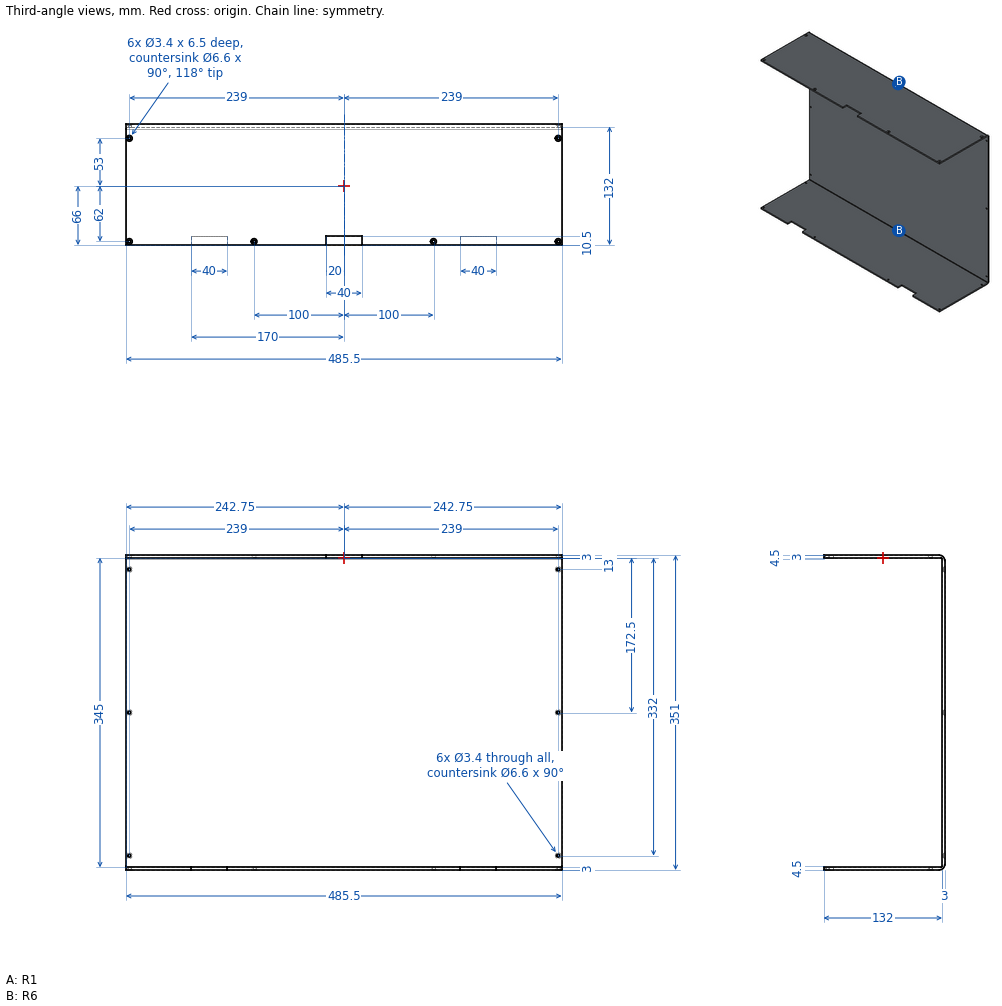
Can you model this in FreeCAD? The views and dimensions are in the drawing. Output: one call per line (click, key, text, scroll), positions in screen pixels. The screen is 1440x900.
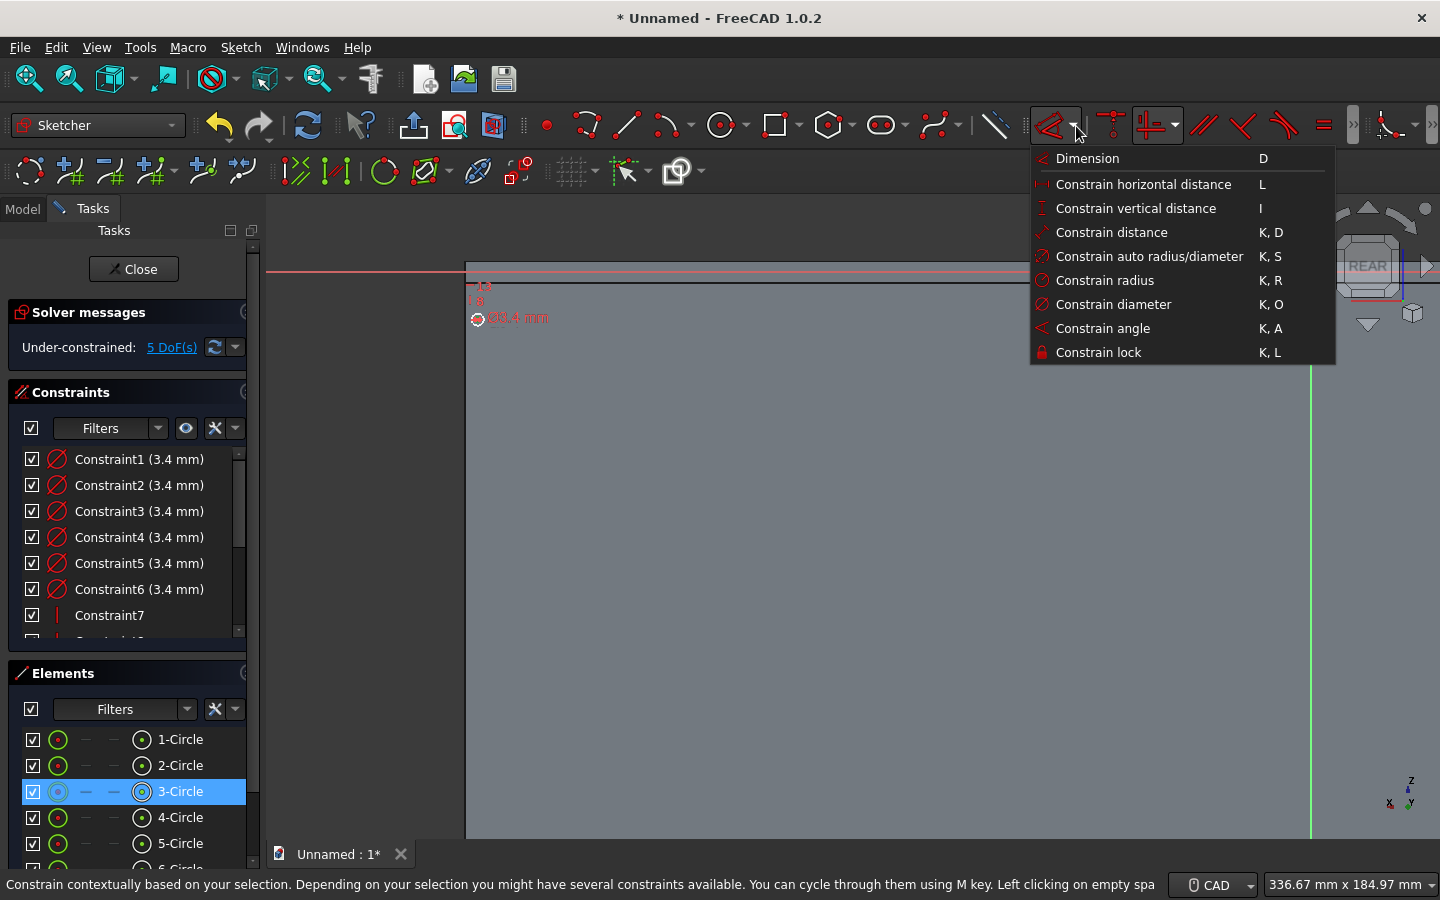
click(1183, 208)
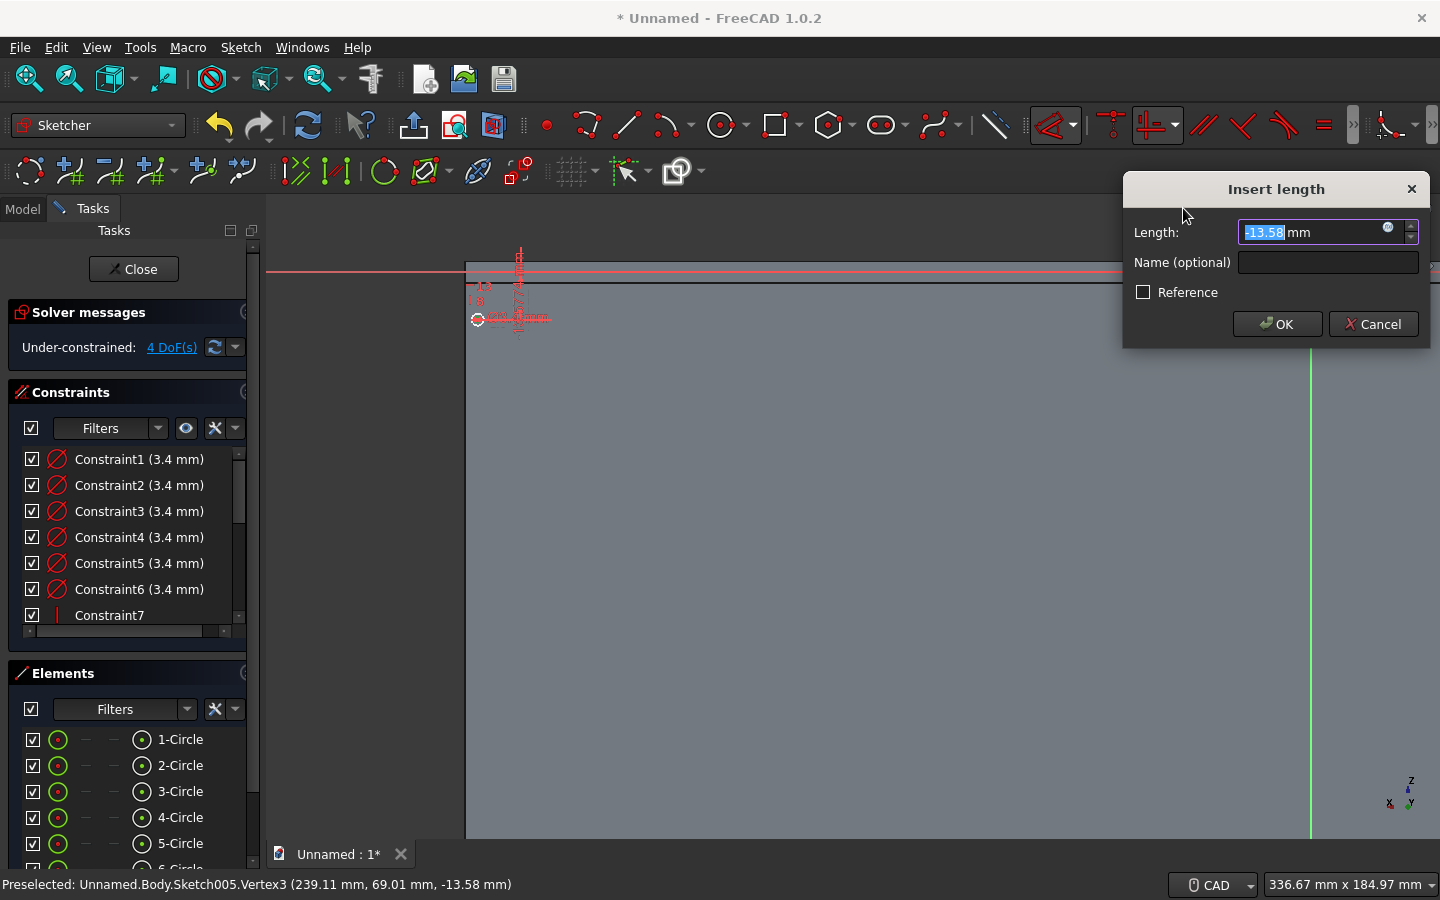
text(-13)
key(Return)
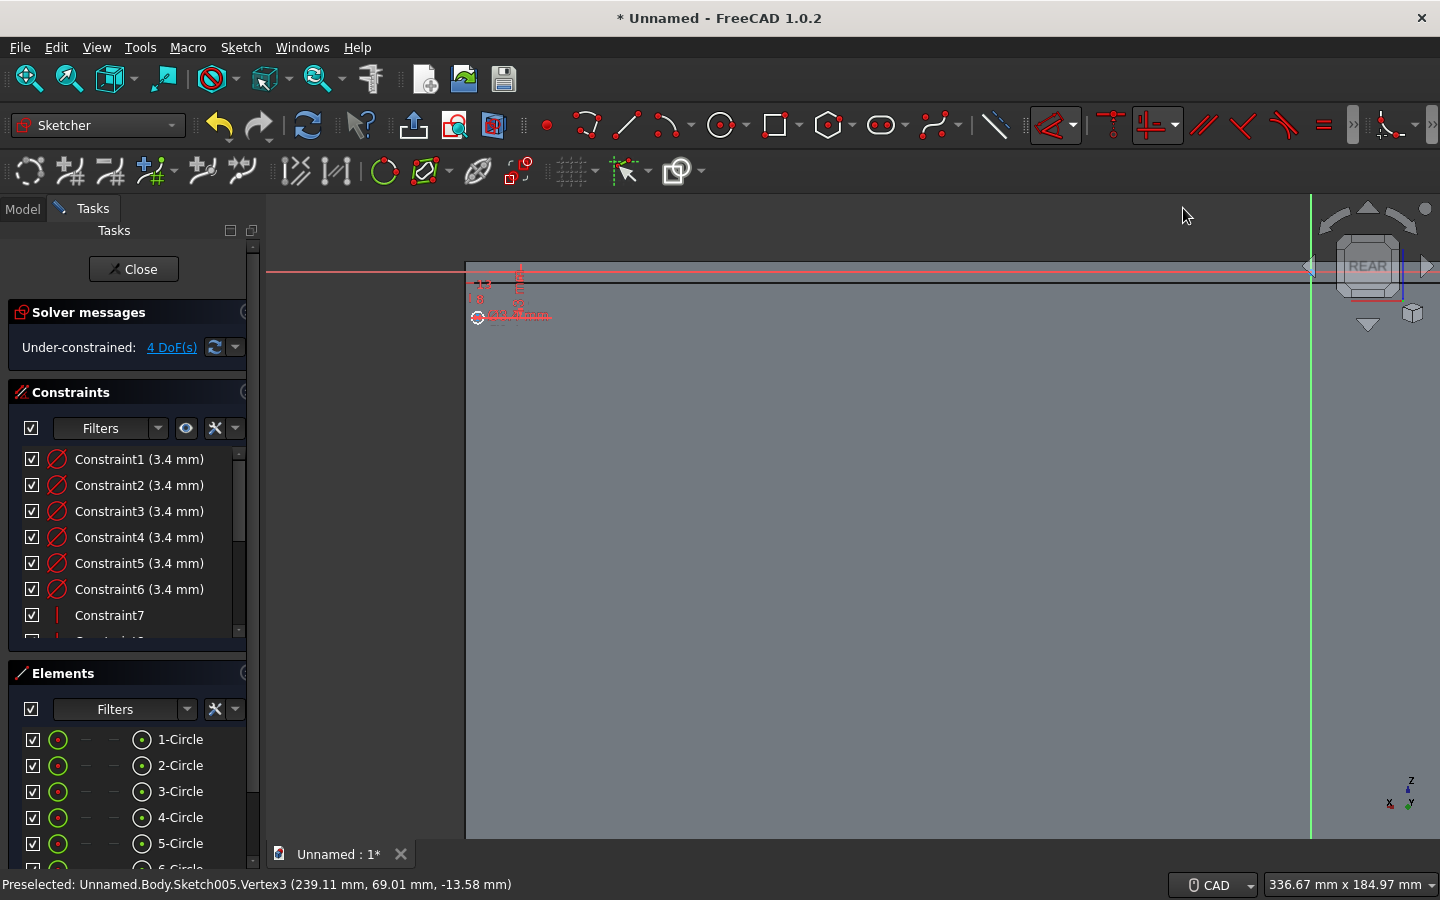
scroll(478, 320, down, 5)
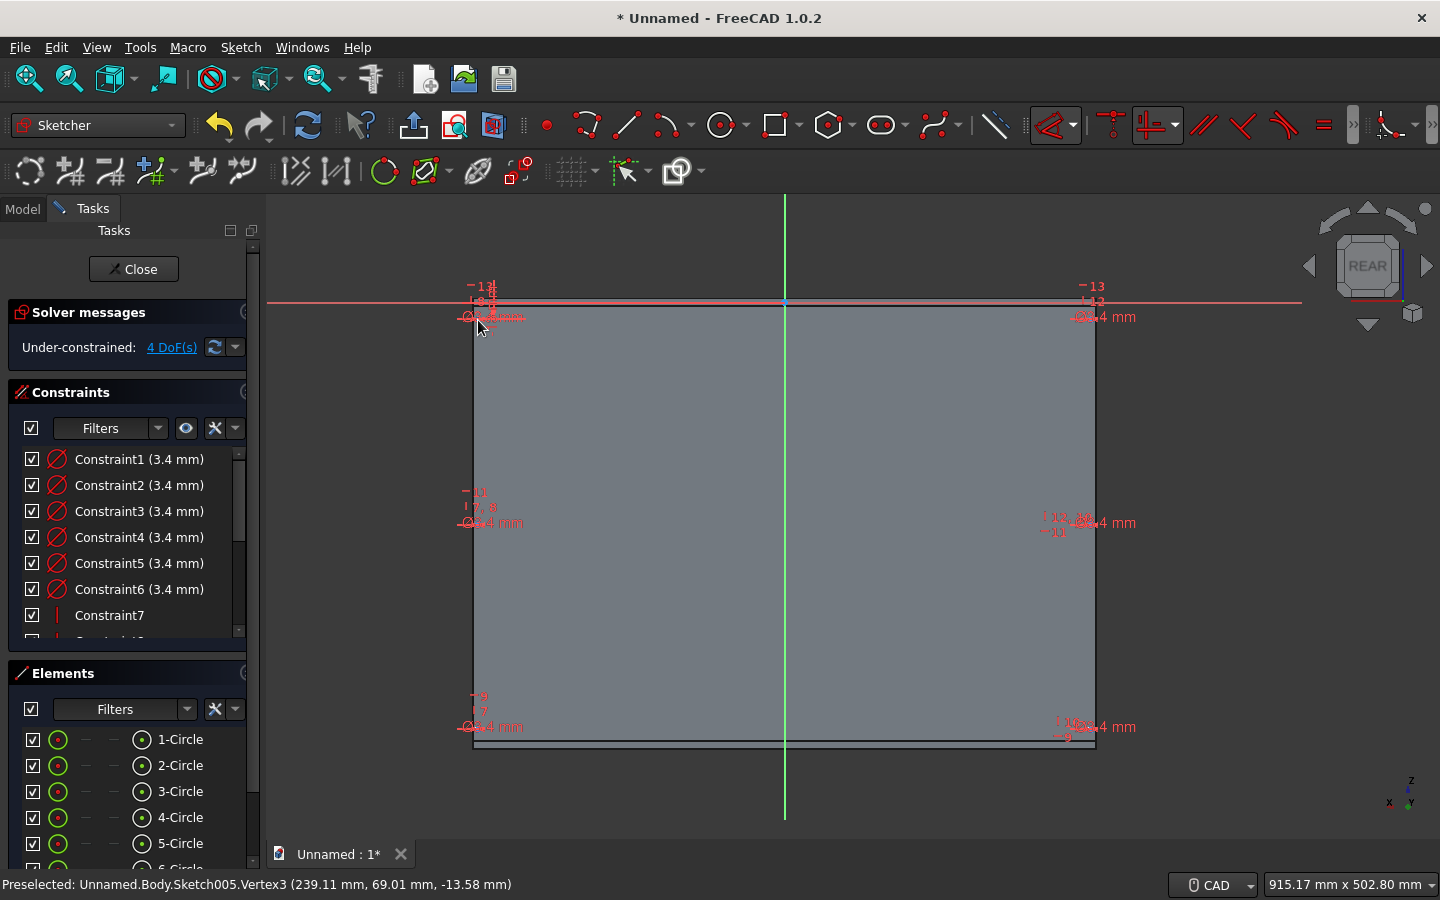
click(478, 729)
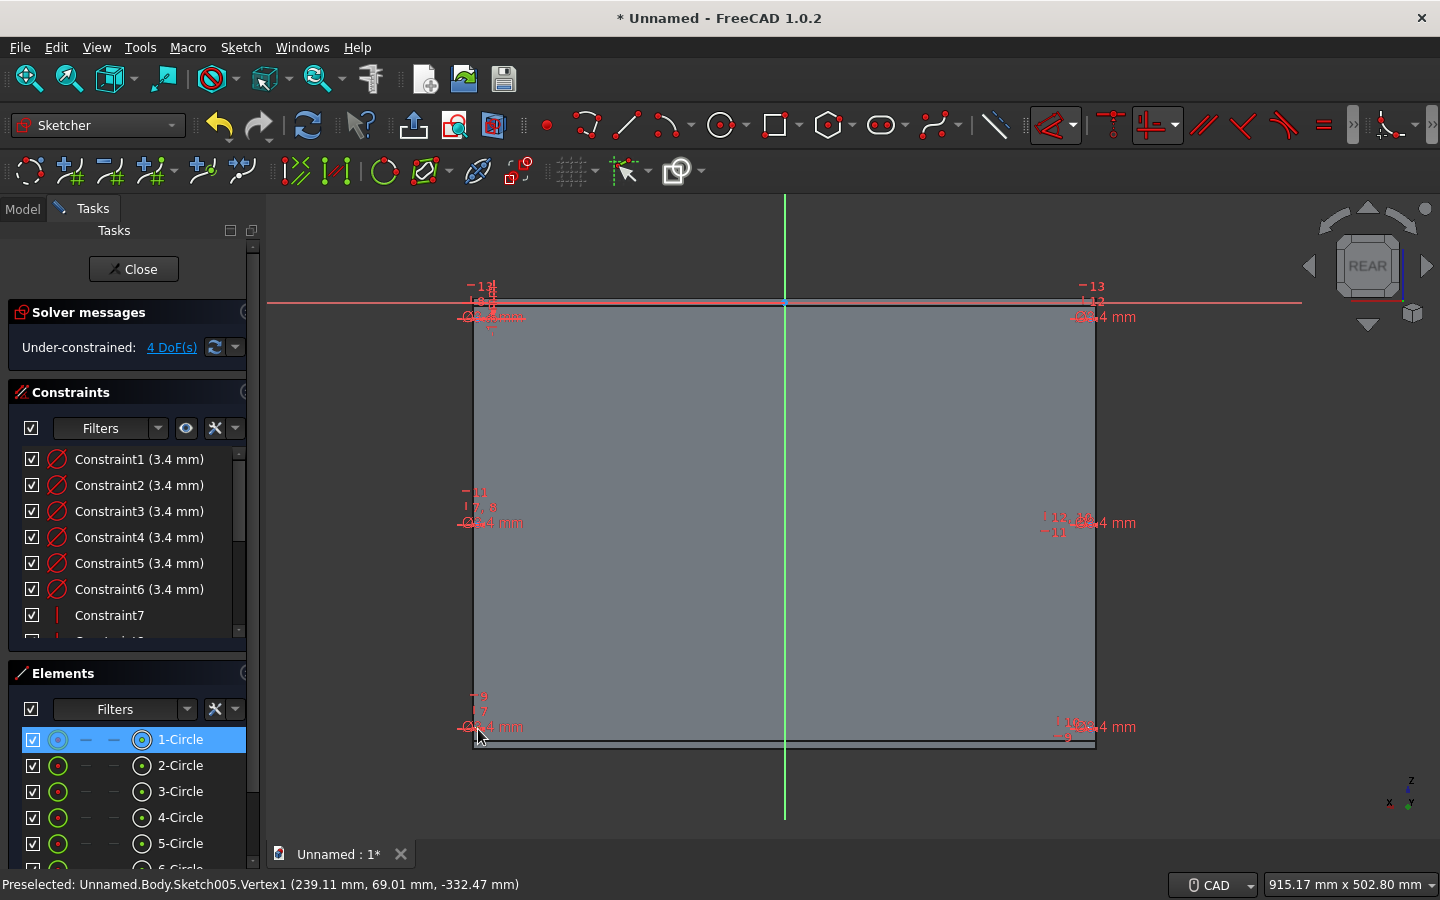
key(l)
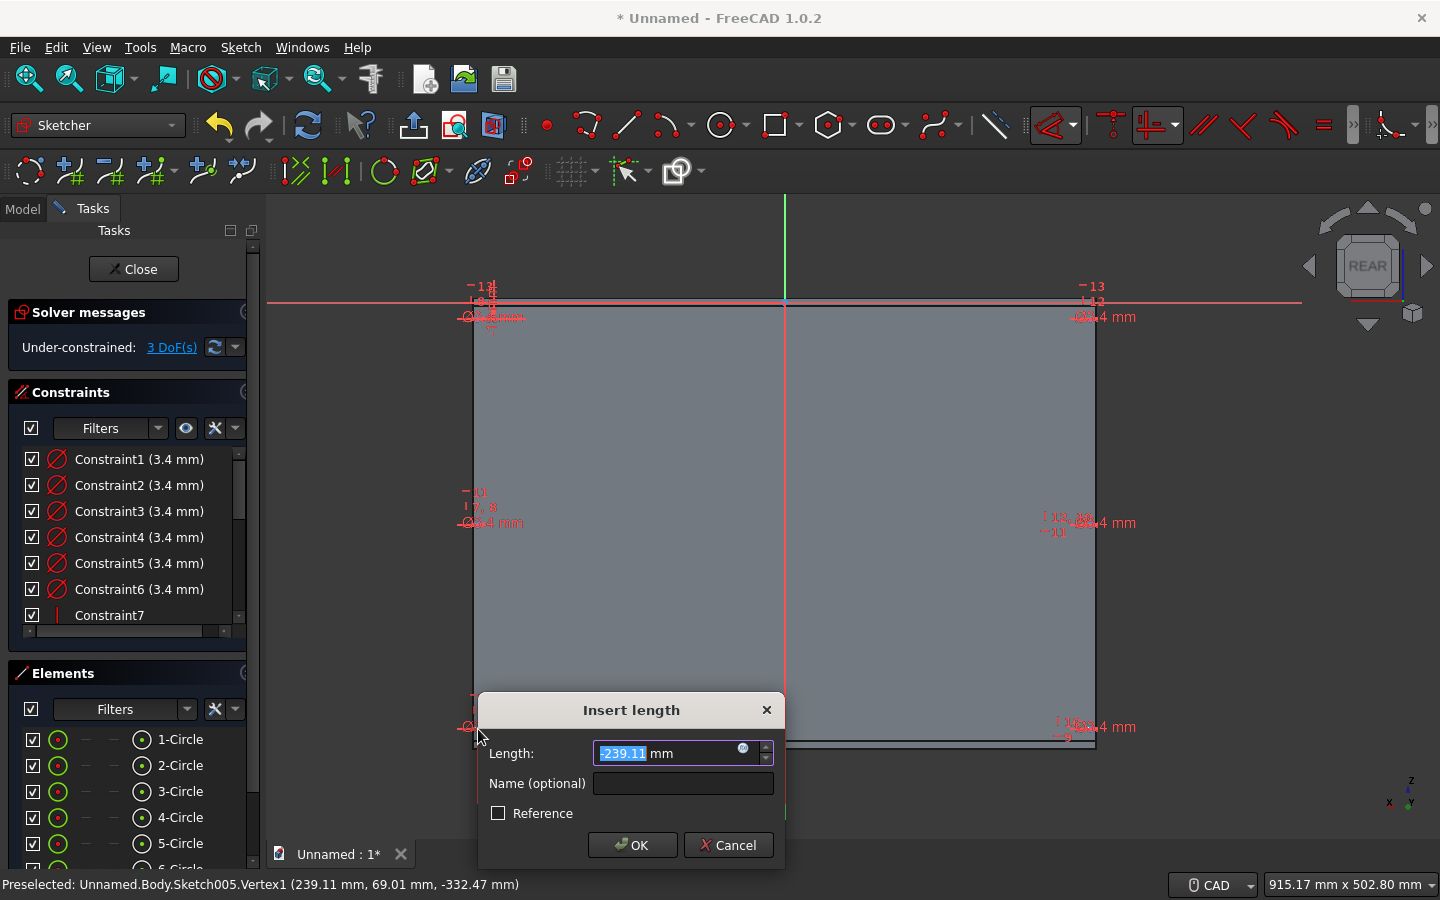
text(-239)
key(Return)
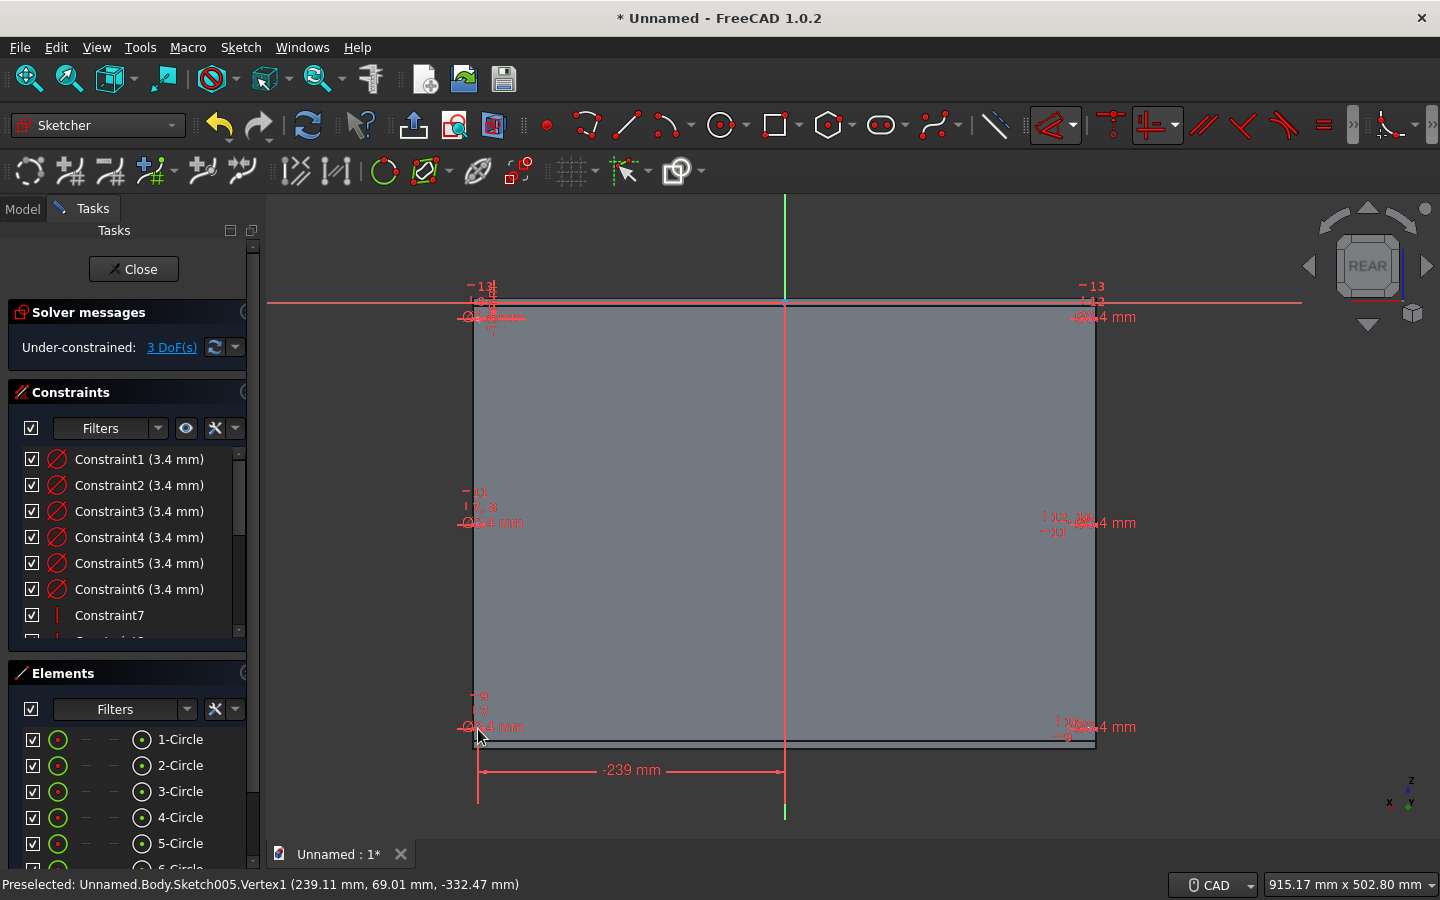
click(478, 729)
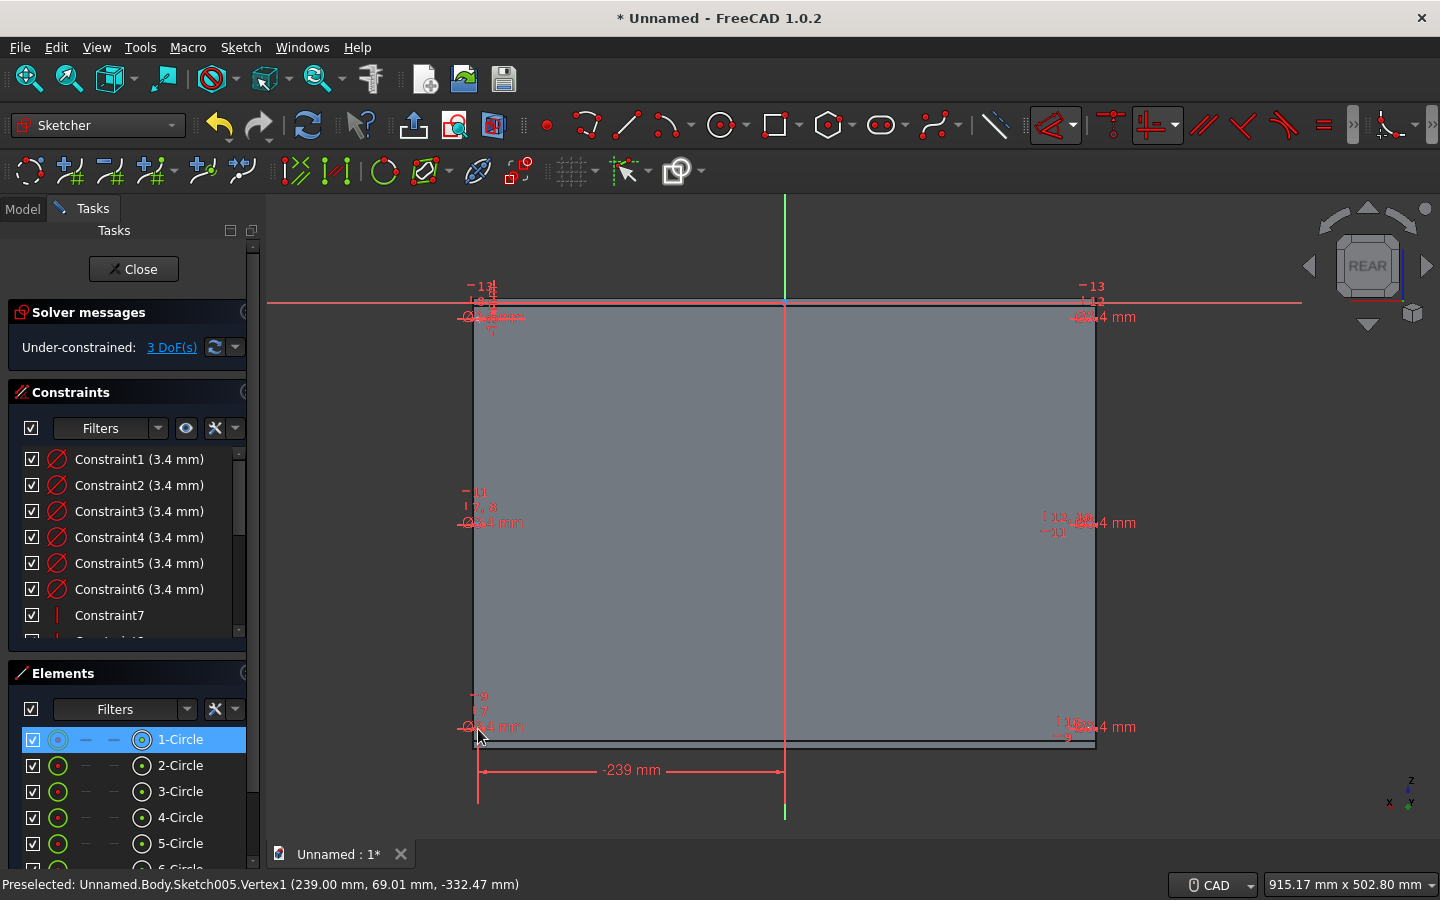
click(1076, 126)